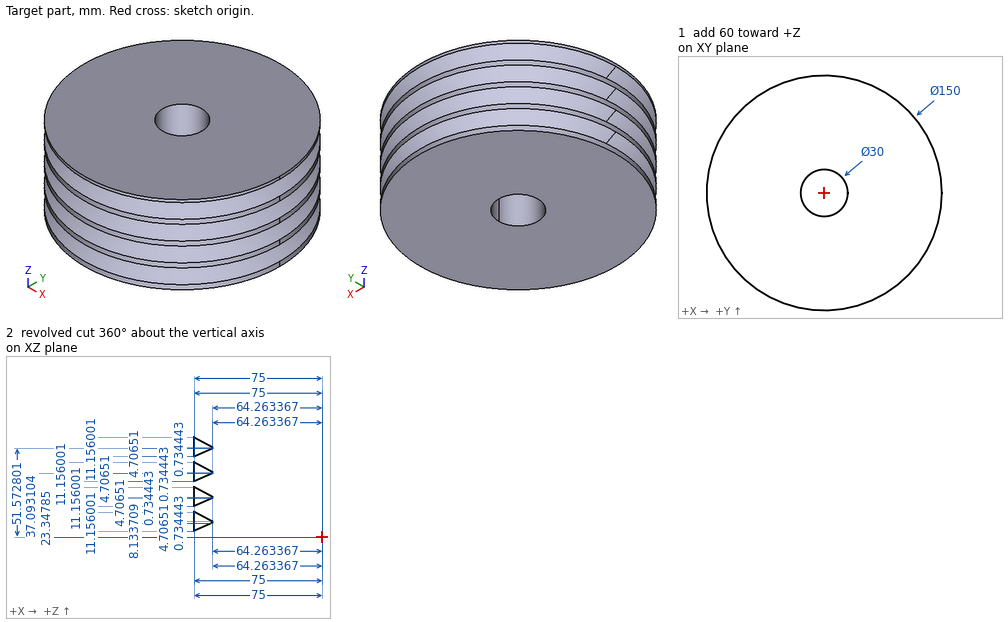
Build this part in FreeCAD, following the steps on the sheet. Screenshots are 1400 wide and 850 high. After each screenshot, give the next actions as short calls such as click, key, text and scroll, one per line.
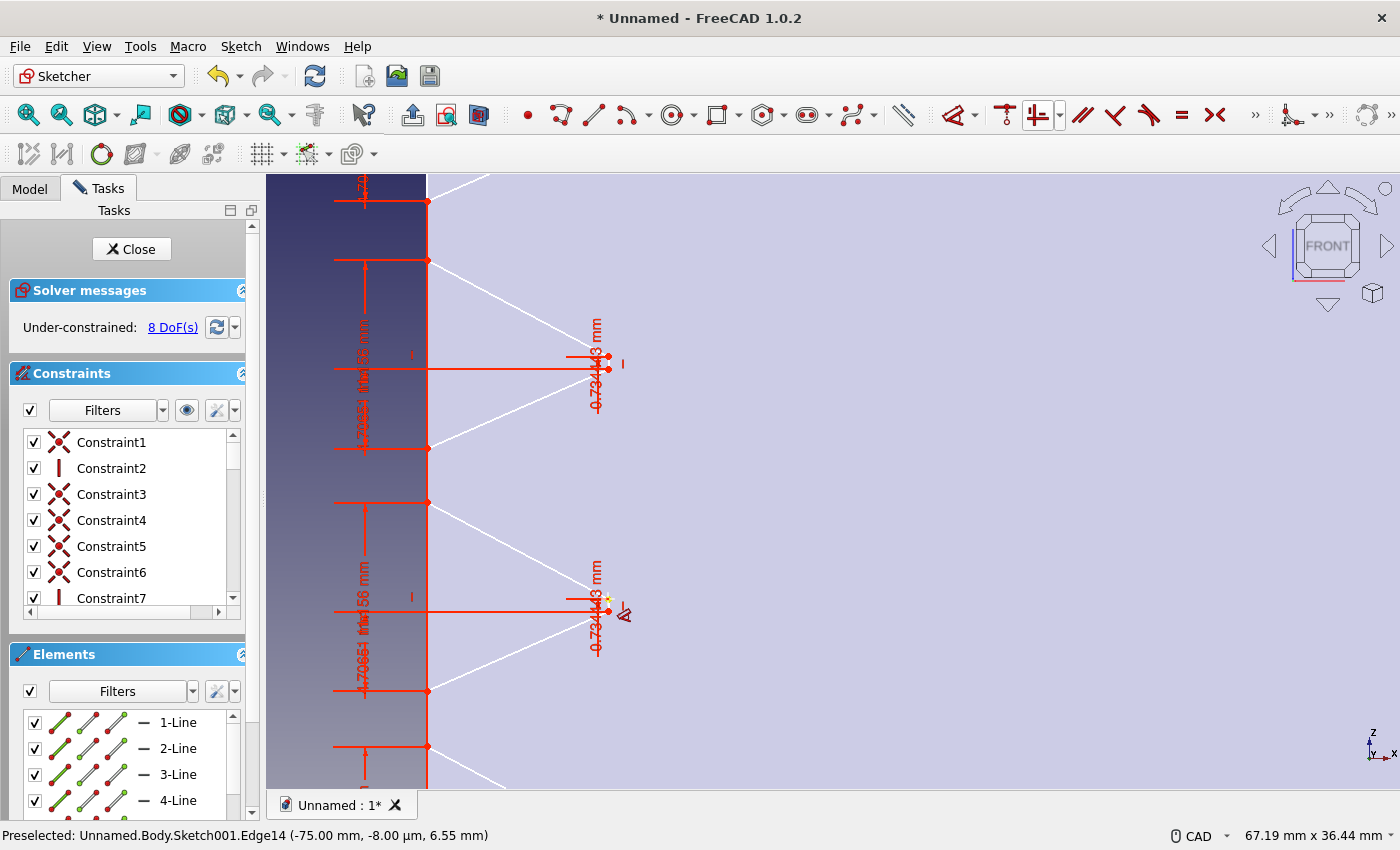
click(609, 599)
click(575, 680)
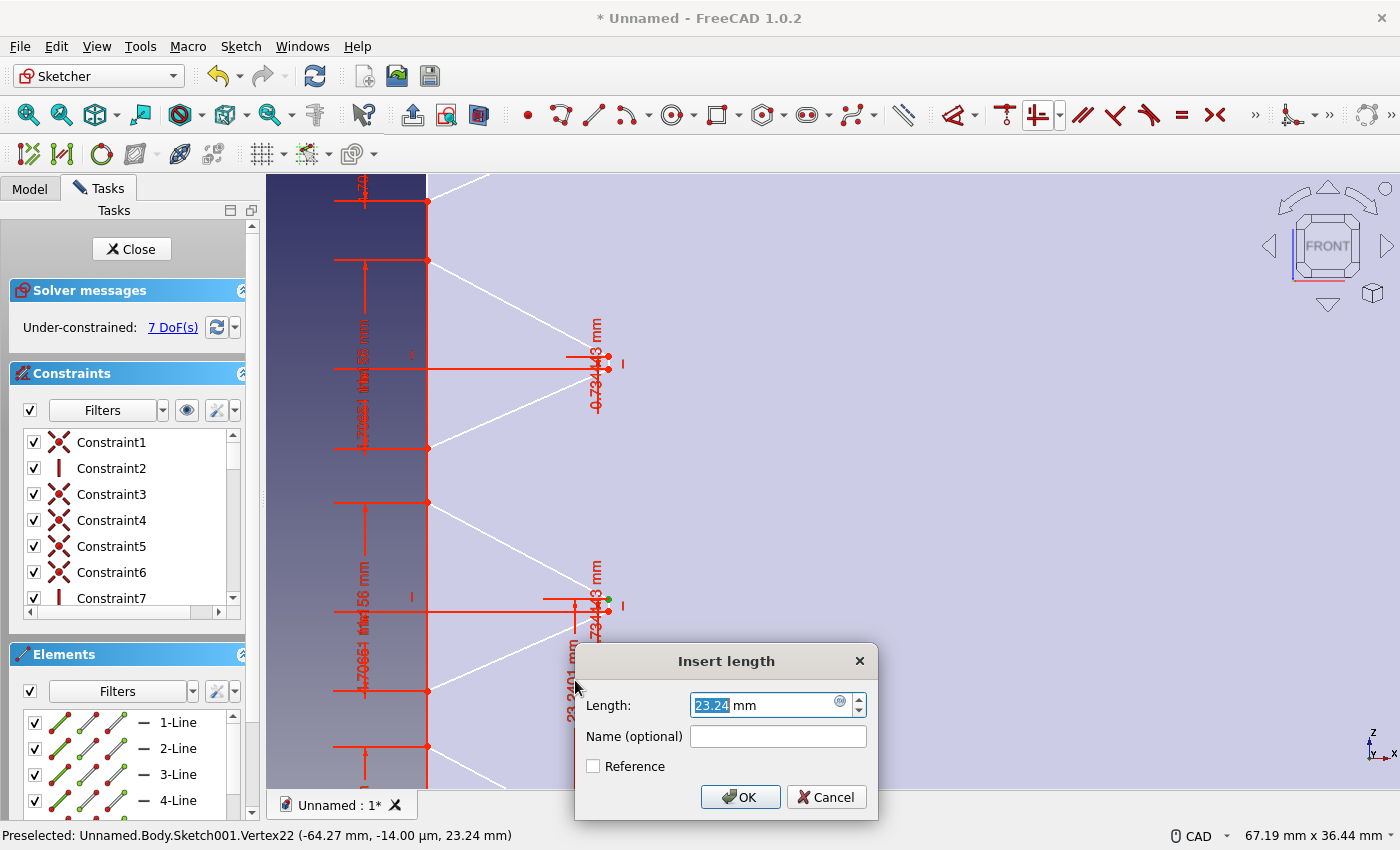
text(23.34785)
key(Return)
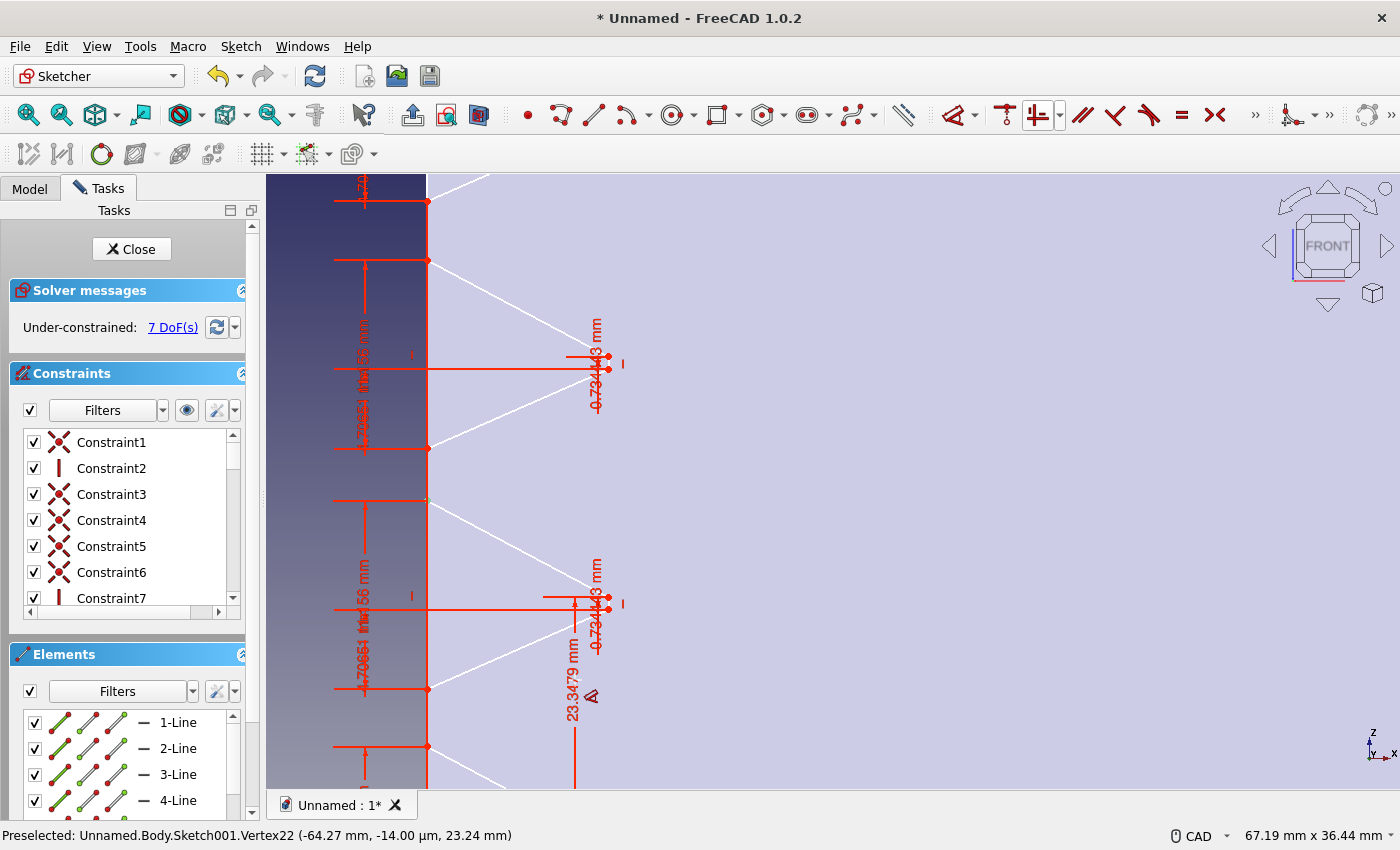
scroll(592, 470, down, 5)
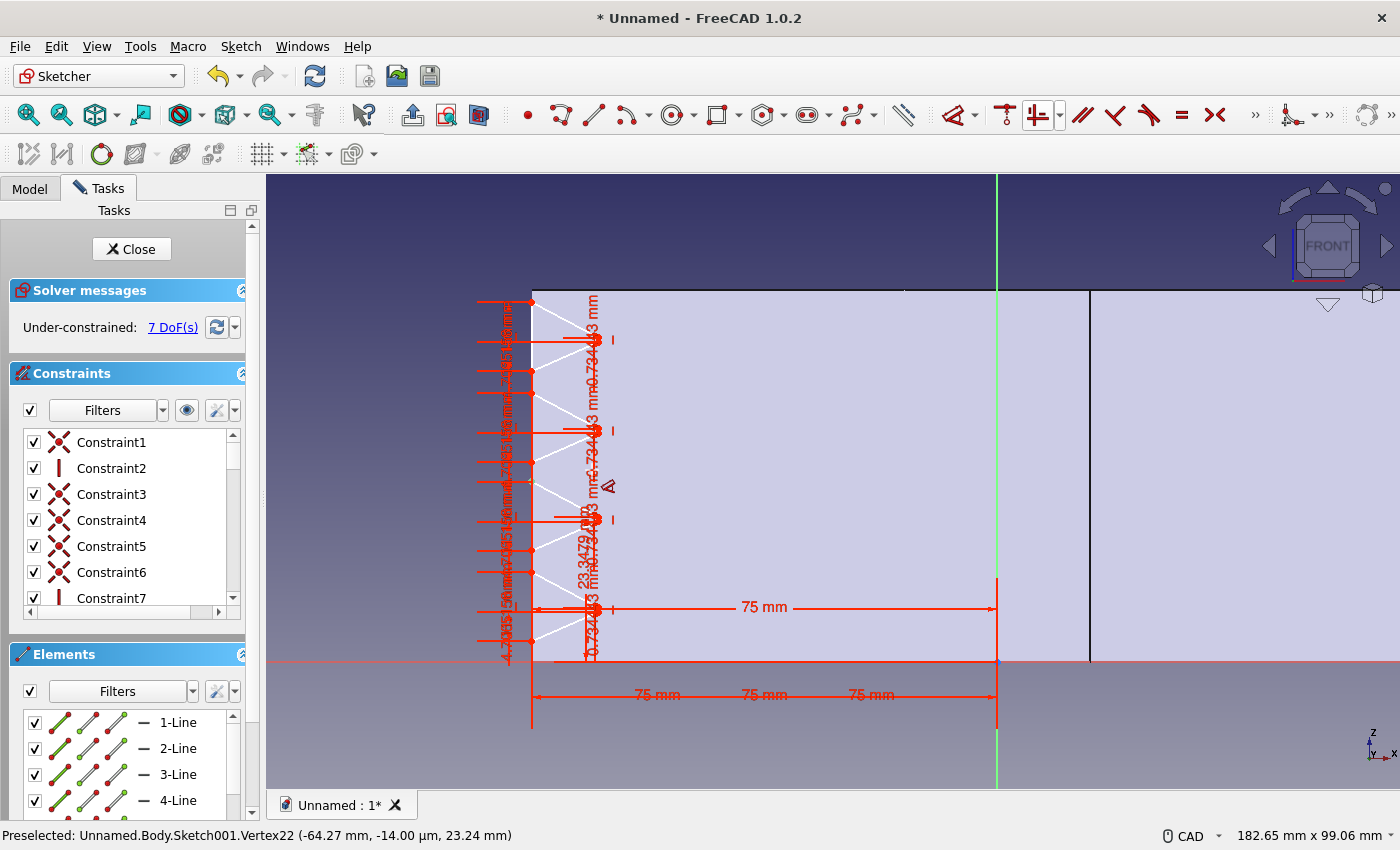
scroll(598, 612, up, 5)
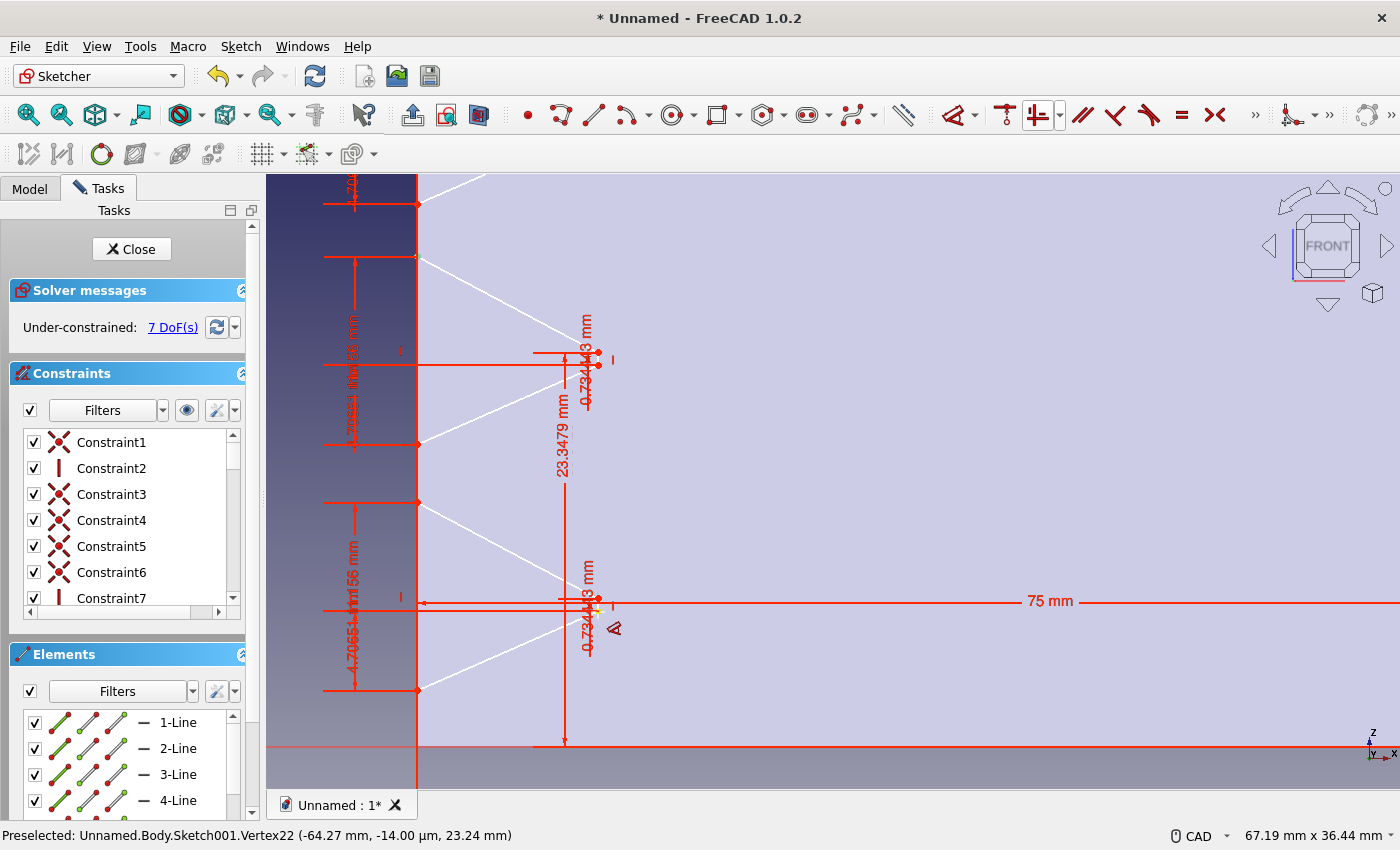
click(598, 611)
click(564, 679)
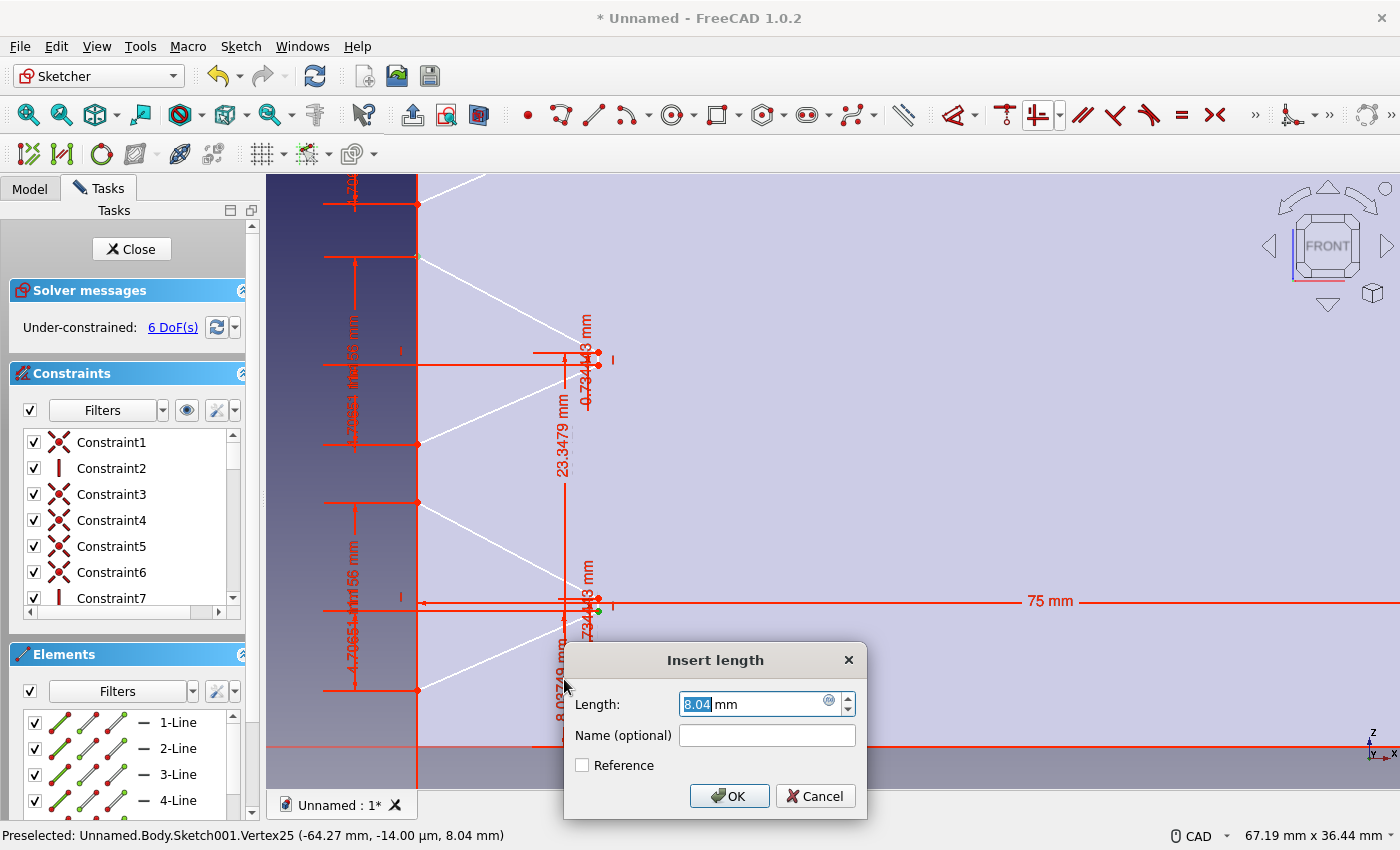
text(8.133709)
key(Return)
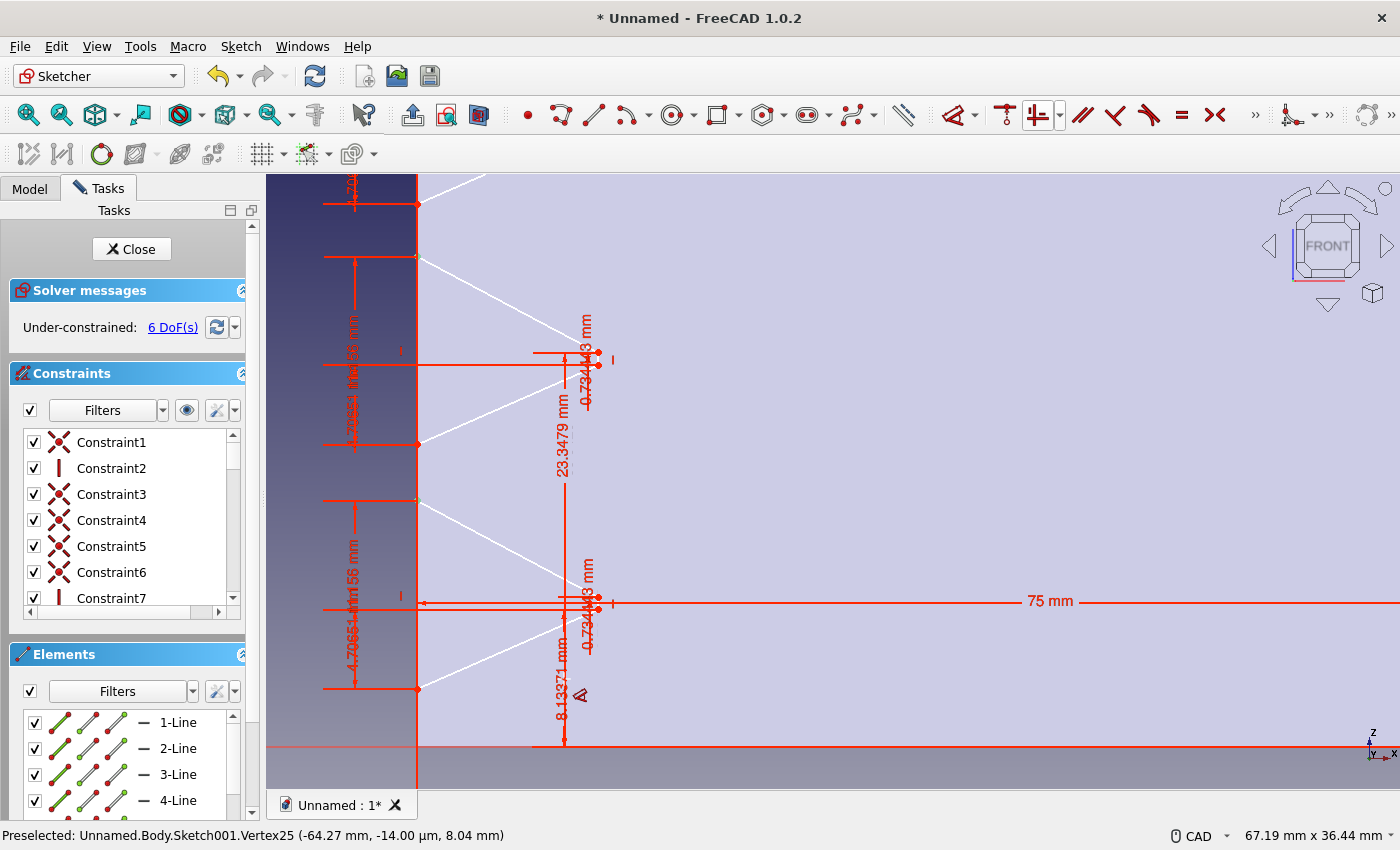
scroll(598, 612, down, 5)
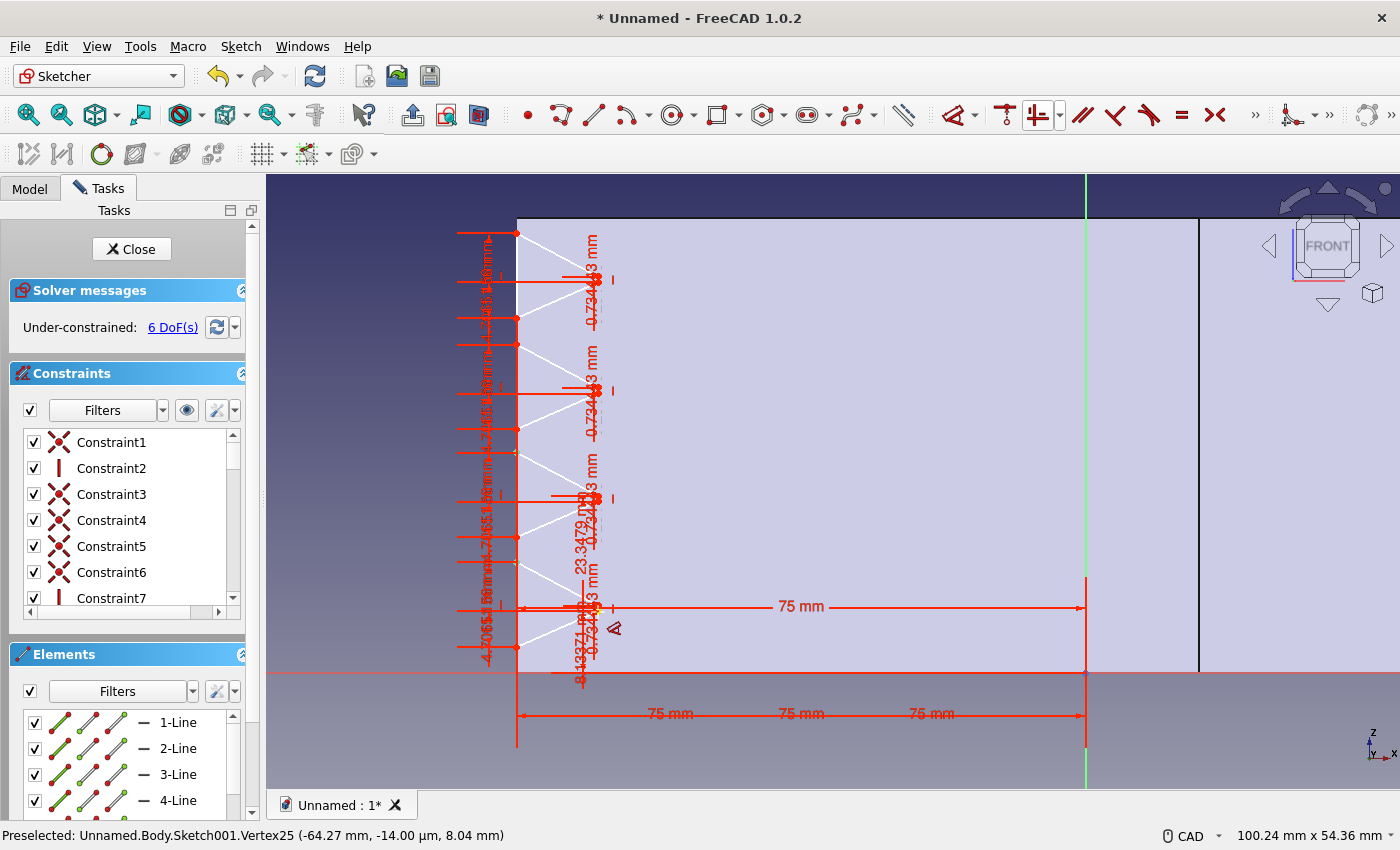
scroll(598, 342, up, 5)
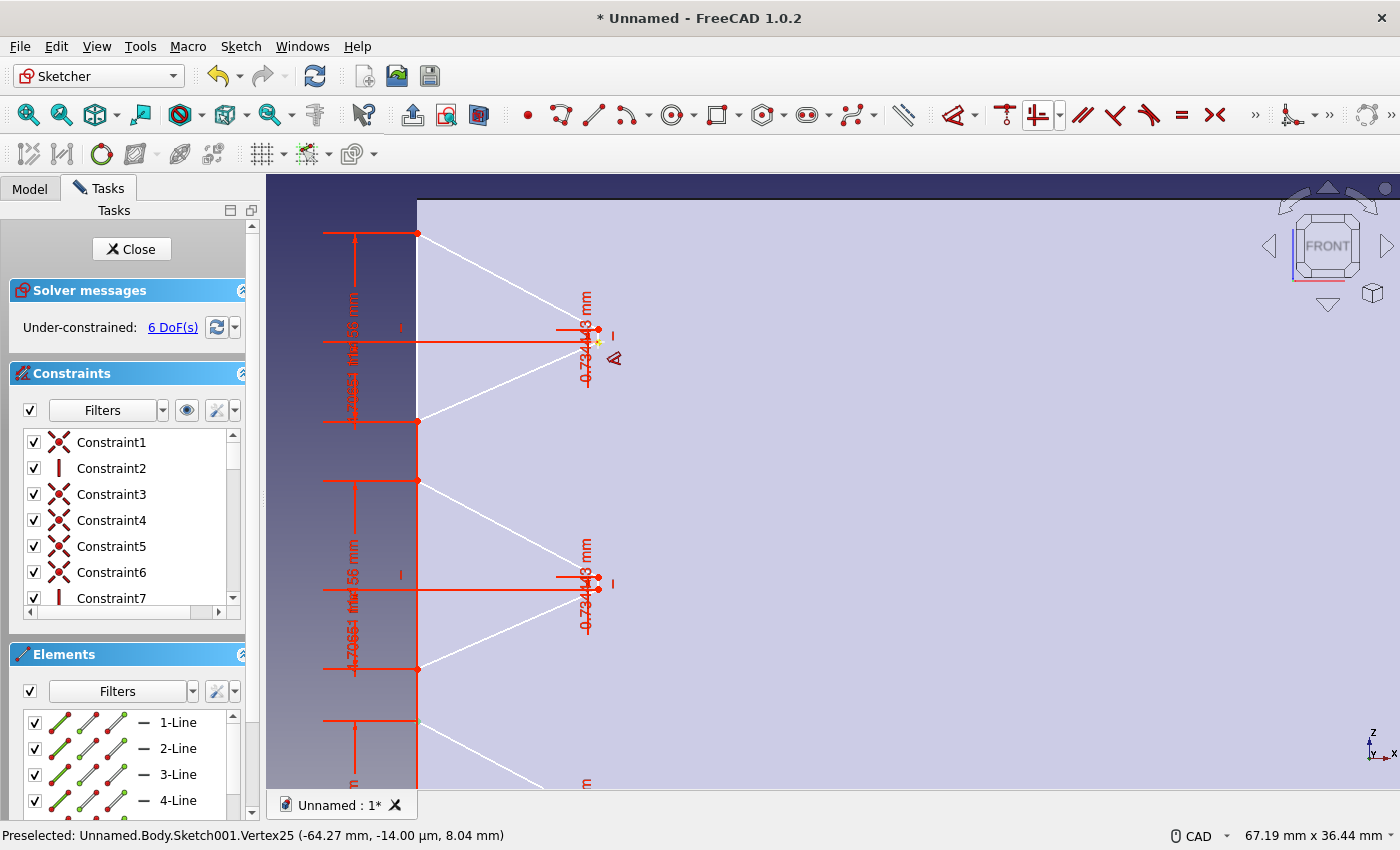
click(598, 342)
click(917, 308)